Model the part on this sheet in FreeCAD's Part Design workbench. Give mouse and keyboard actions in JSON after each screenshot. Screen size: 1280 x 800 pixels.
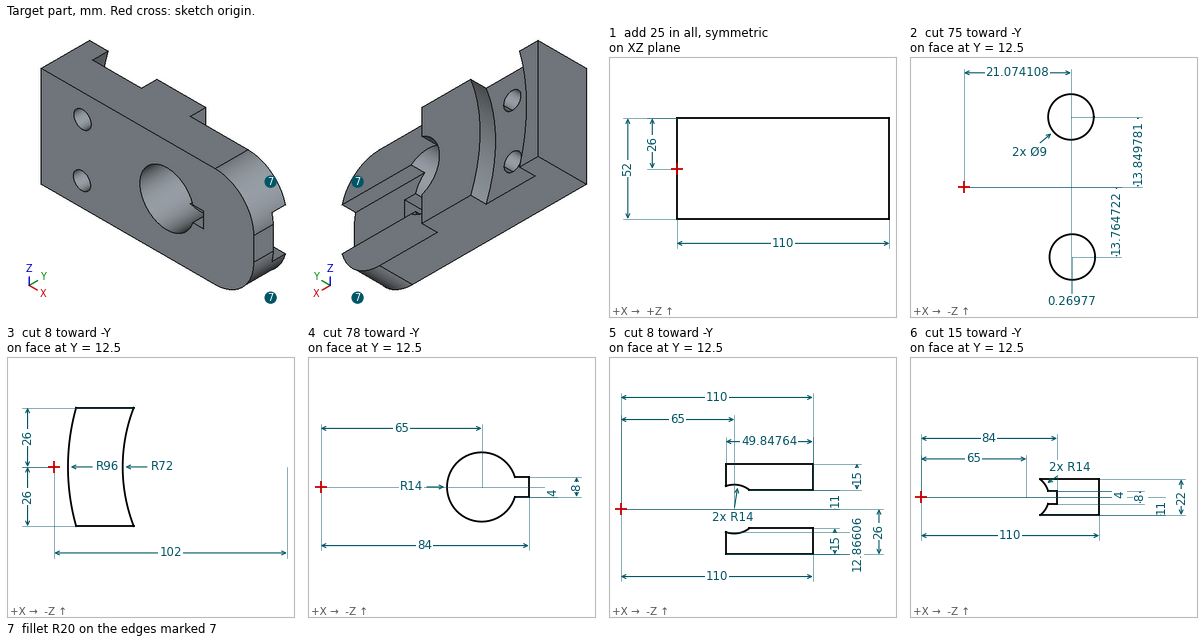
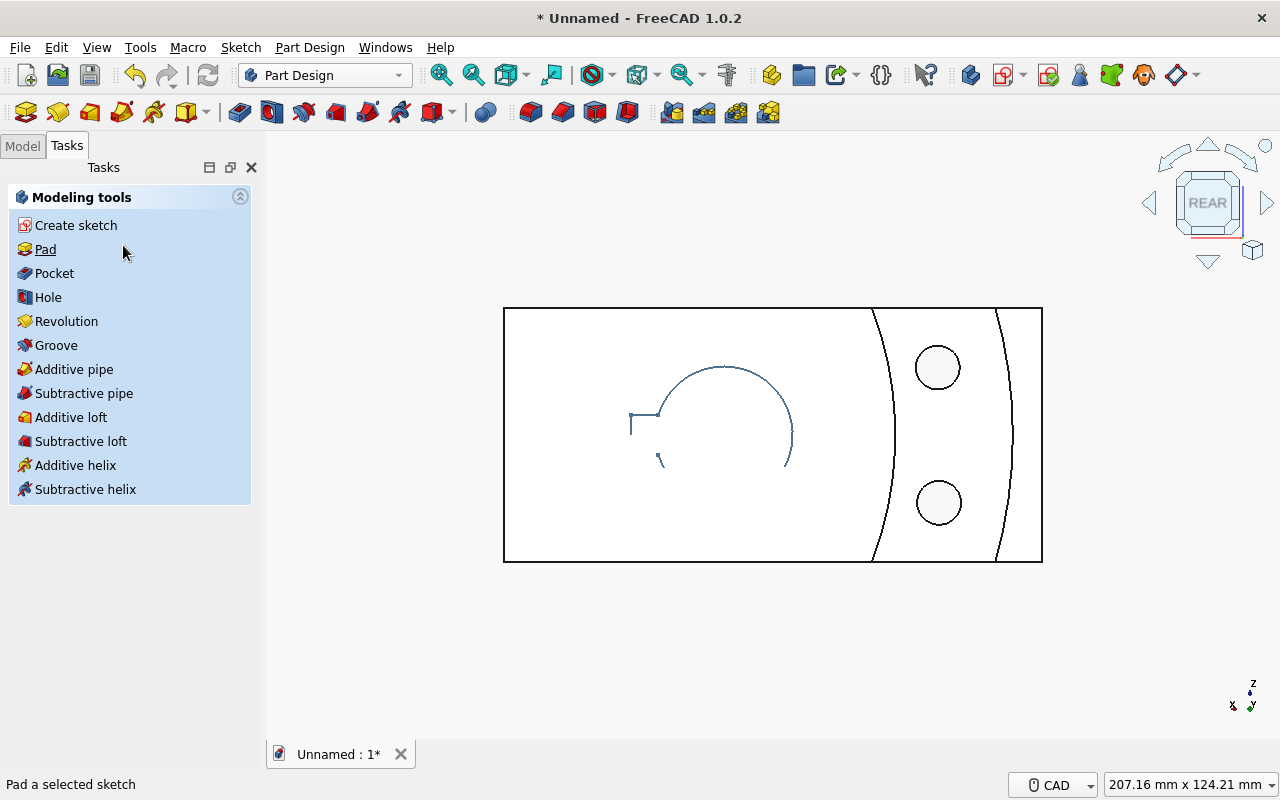
{"action": "left_click", "coordinate": [240, 112]}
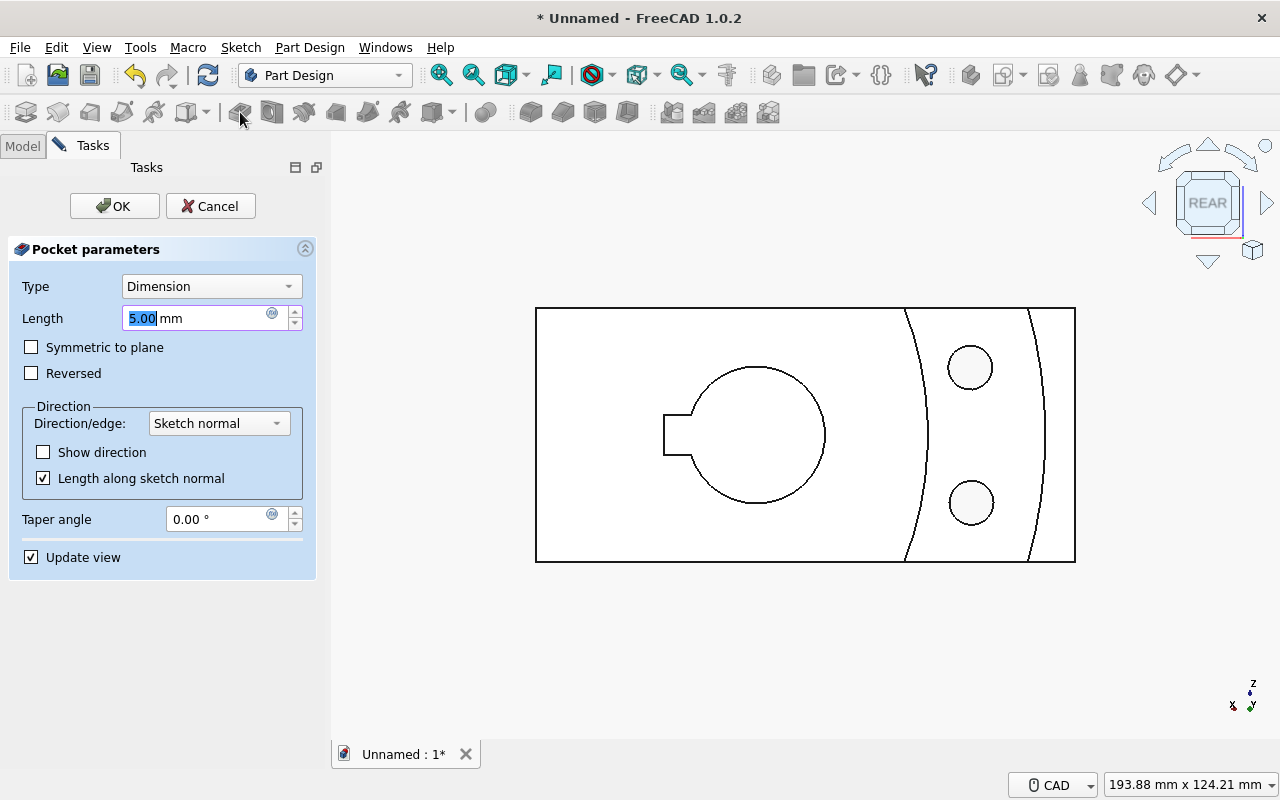
{"action": "type", "text": "78"}
{"action": "key", "text": "Tab"}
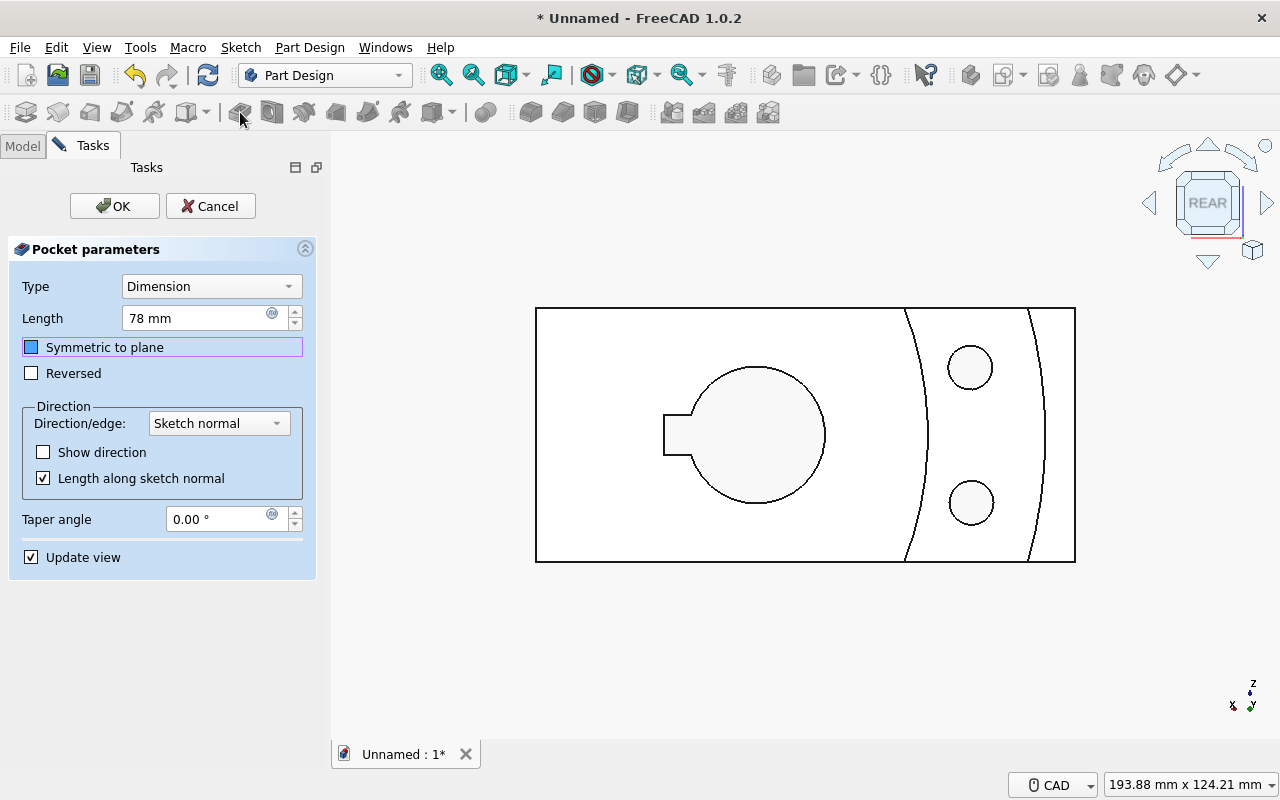
{"action": "left_click", "coordinate": [115, 206]}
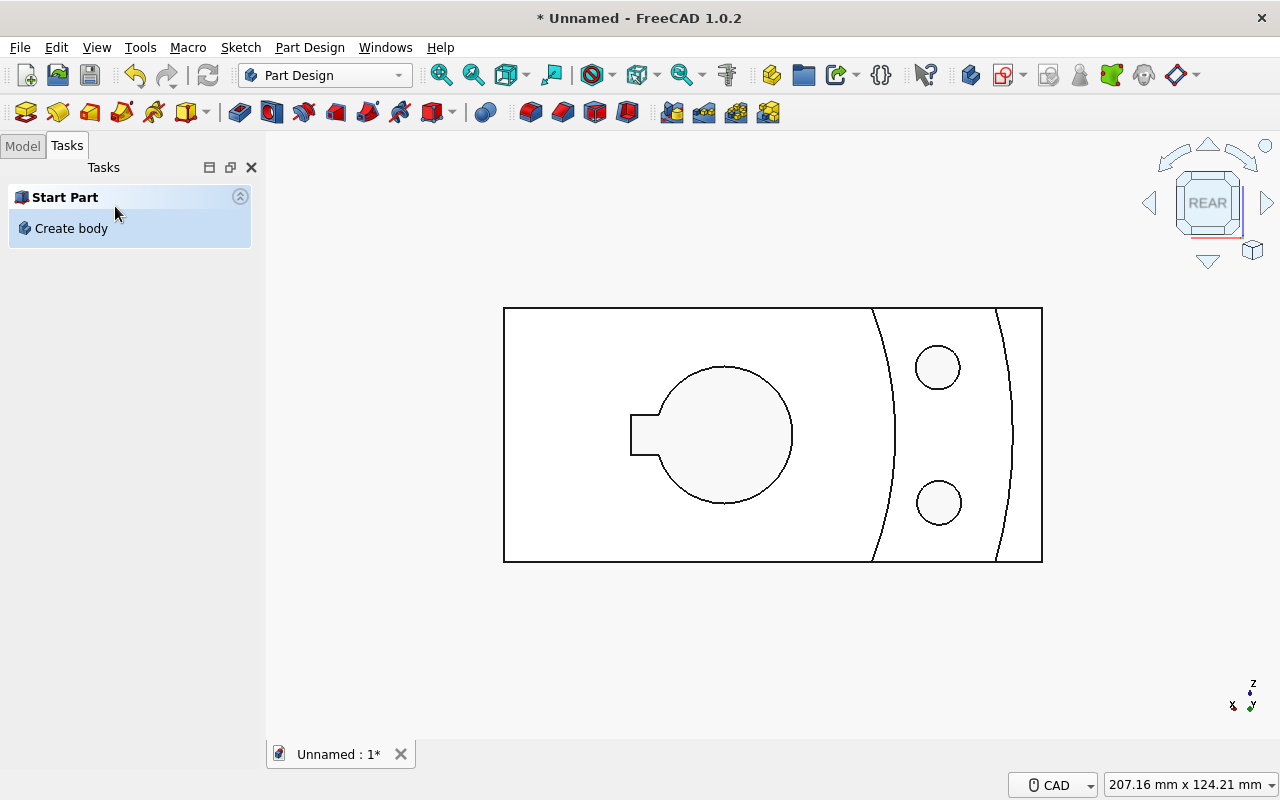
{"action": "left_click", "coordinate": [588, 361]}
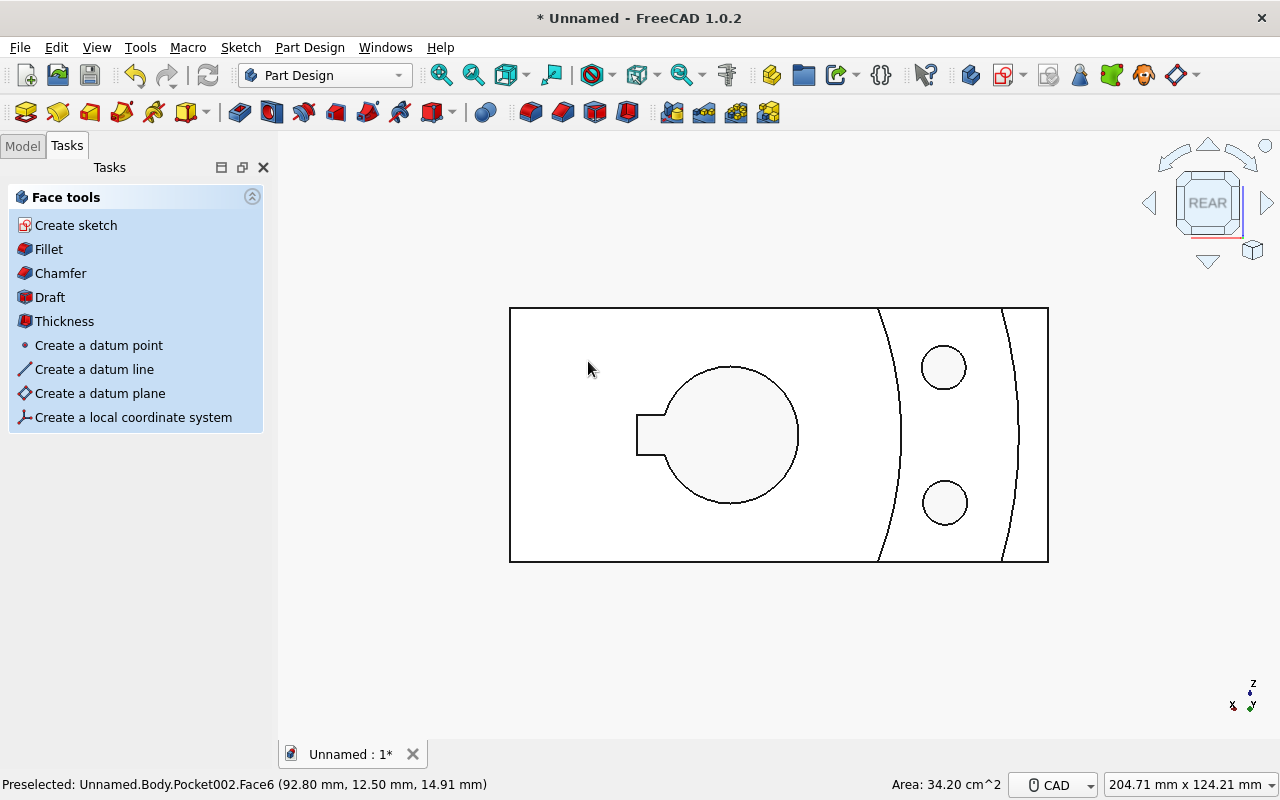
{"action": "left_click", "coordinate": [1004, 76]}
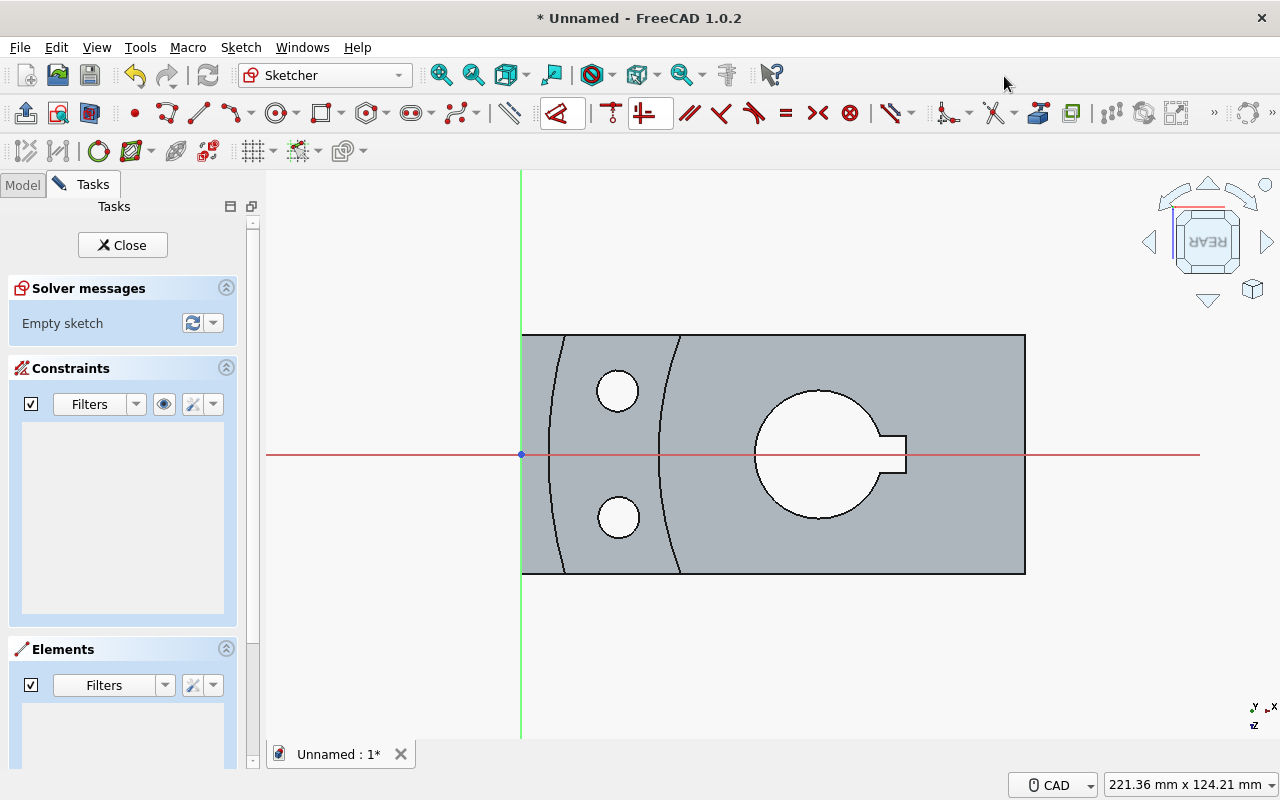
{"action": "left_click", "coordinate": [168, 114]}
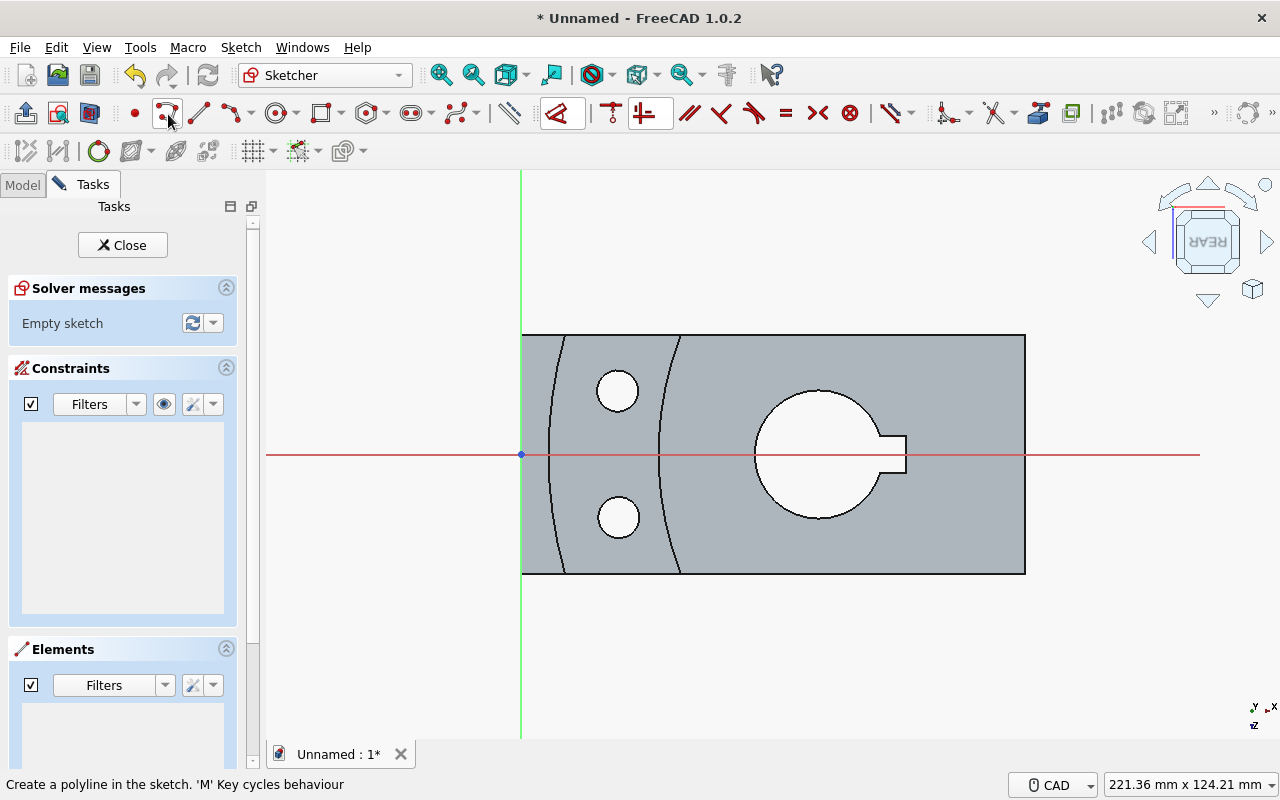
{"action": "left_click", "coordinate": [858, 404]}
{"action": "left_click", "coordinate": [1025, 404]}
{"action": "left_click", "coordinate": [1025, 335]}
{"action": "left_click", "coordinate": [797, 335]}
{"action": "left_click", "coordinate": [797, 394]}
{"action": "right_click", "coordinate": [797, 394]}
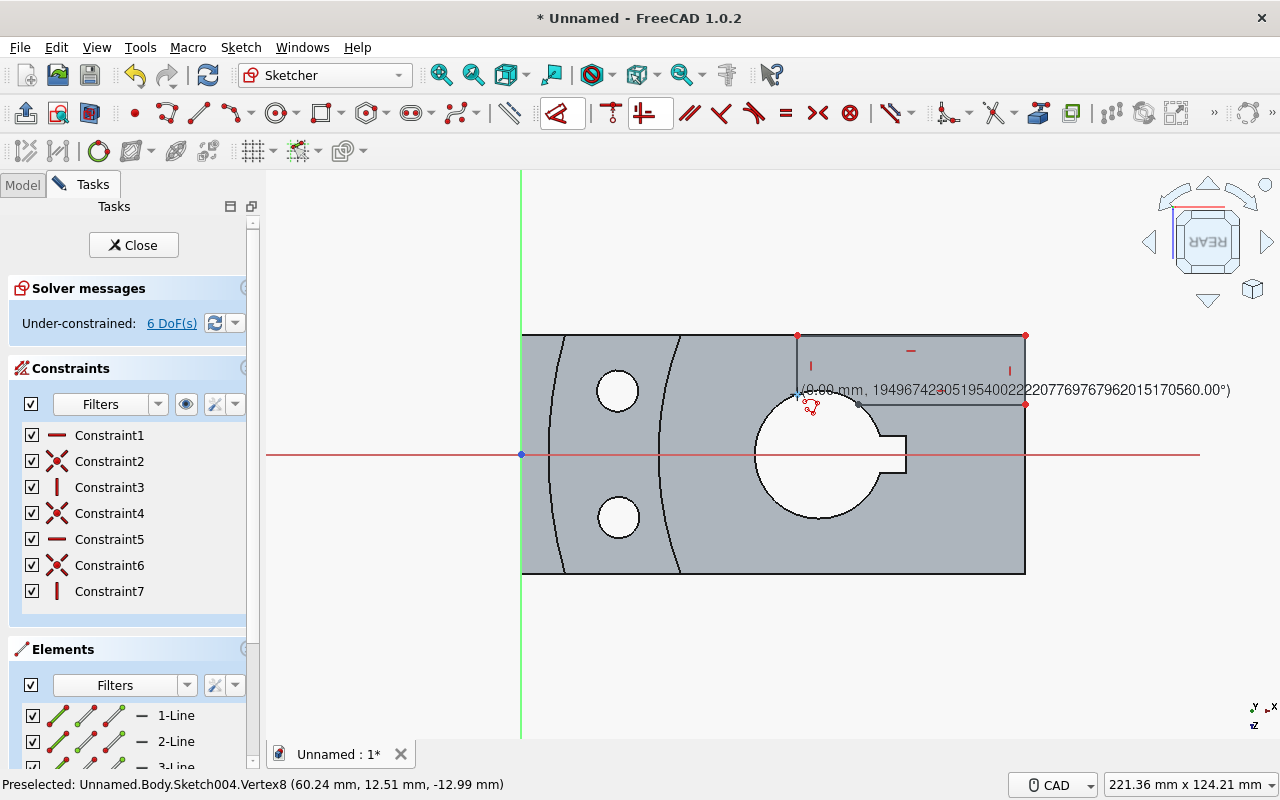
{"action": "left_click", "coordinate": [232, 114]}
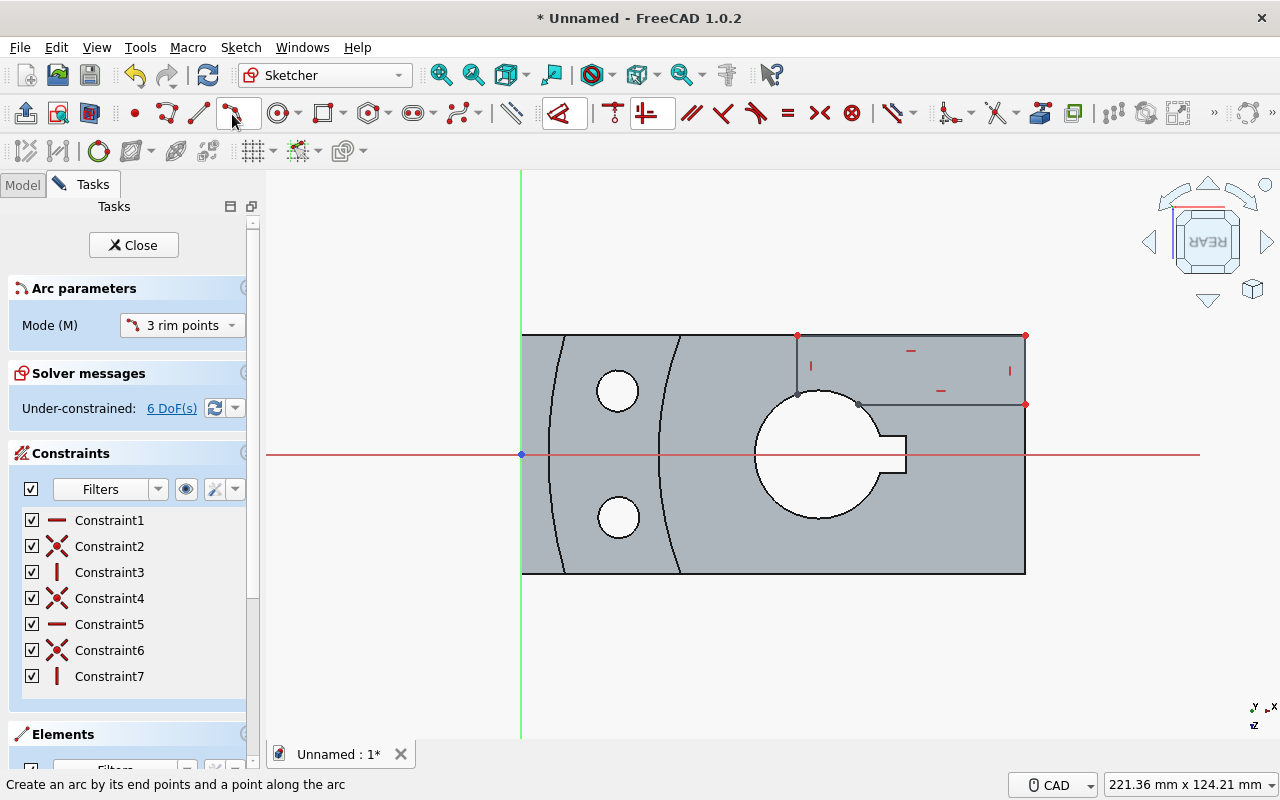
{"action": "left_click", "coordinate": [797, 395]}
{"action": "left_click", "coordinate": [858, 405]}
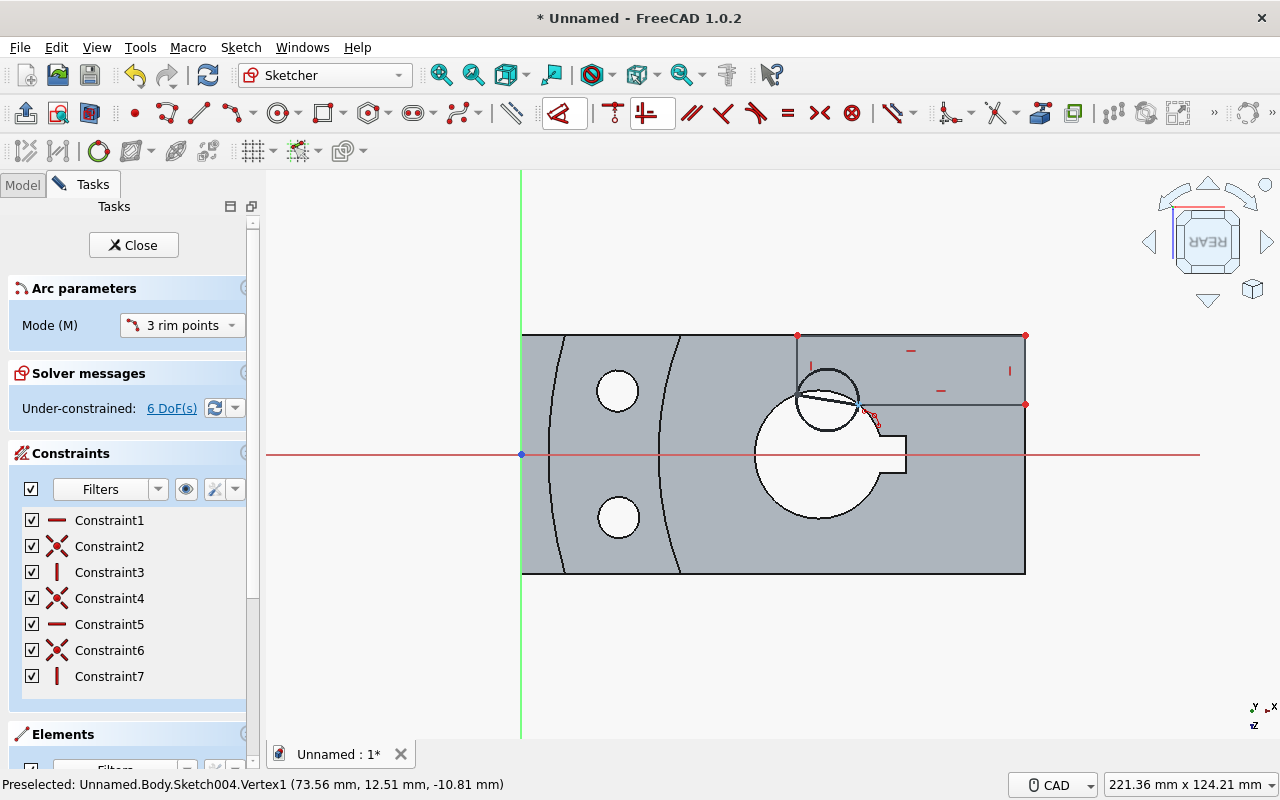
{"action": "scroll", "coordinate": [829, 391], "scroll_direction": "up", "scroll_amount": 4}